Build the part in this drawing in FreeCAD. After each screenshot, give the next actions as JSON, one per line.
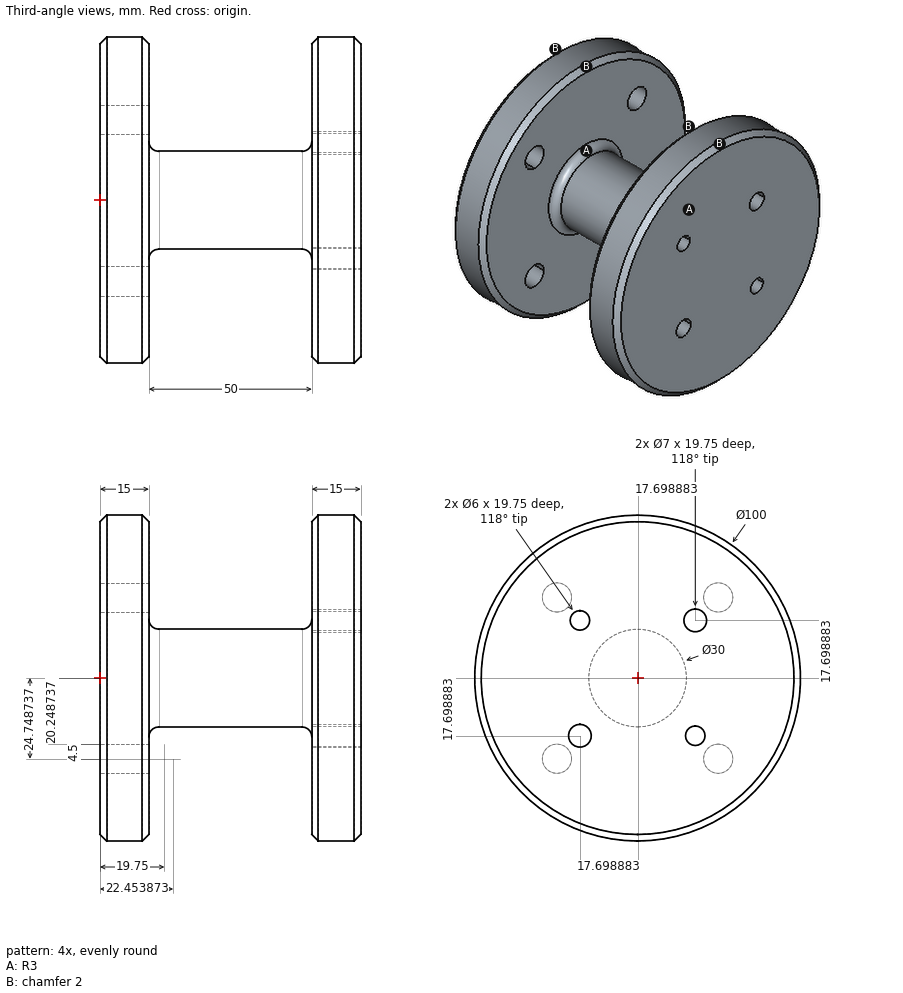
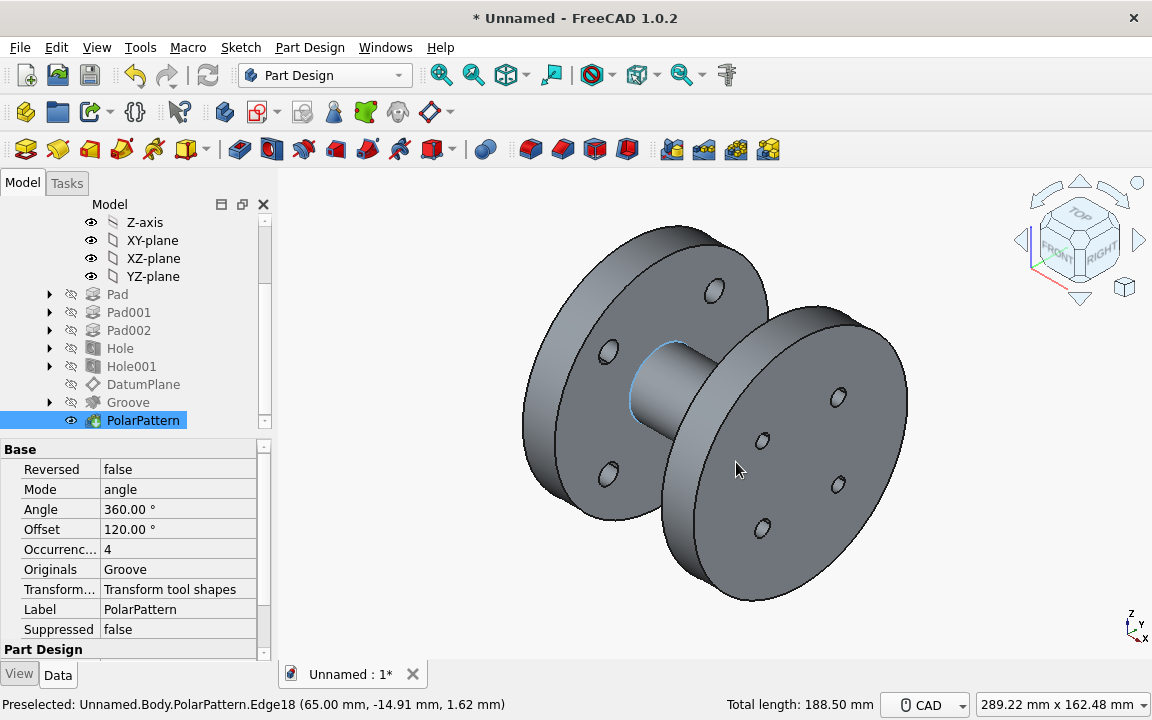
{"action": "left_click", "coordinate": [532, 150]}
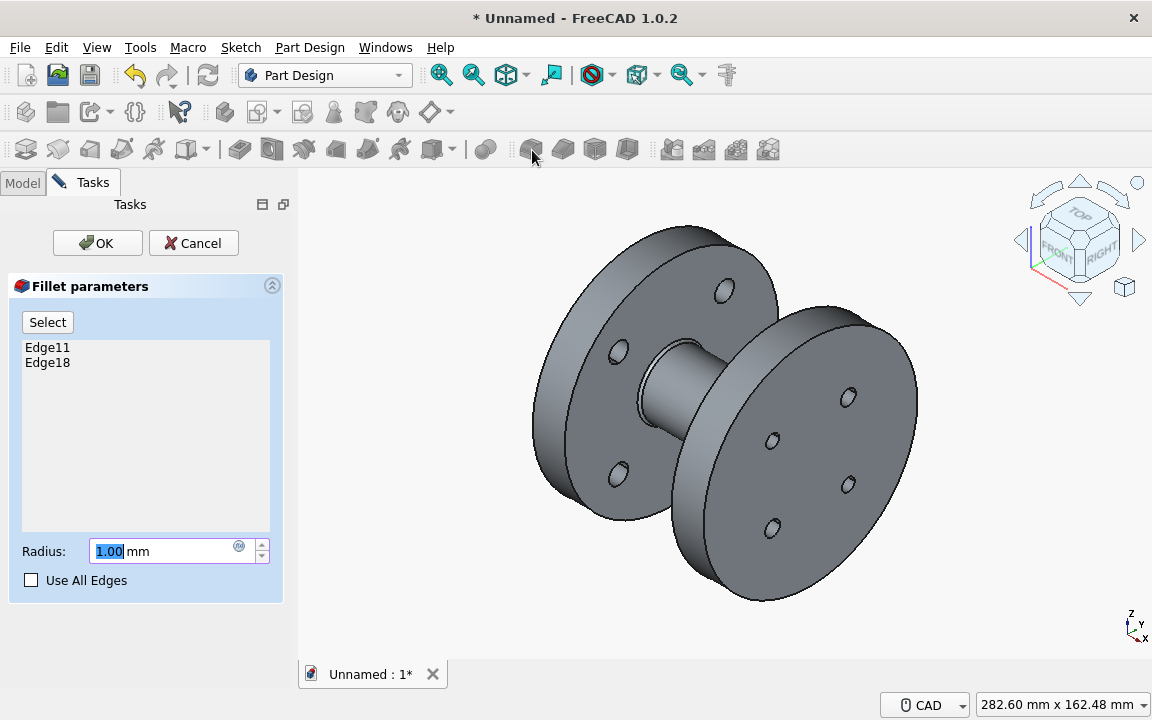
{"action": "type", "text": "3"}
{"action": "key", "text": "Tab"}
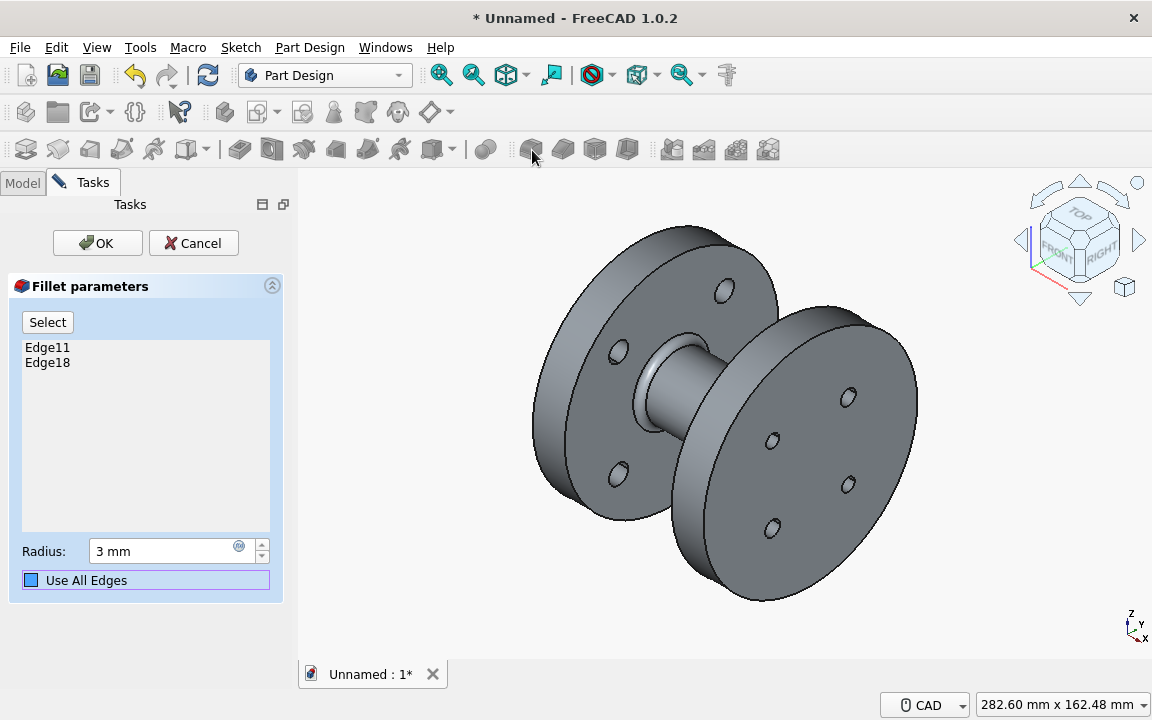
{"action": "left_click", "coordinate": [98, 243]}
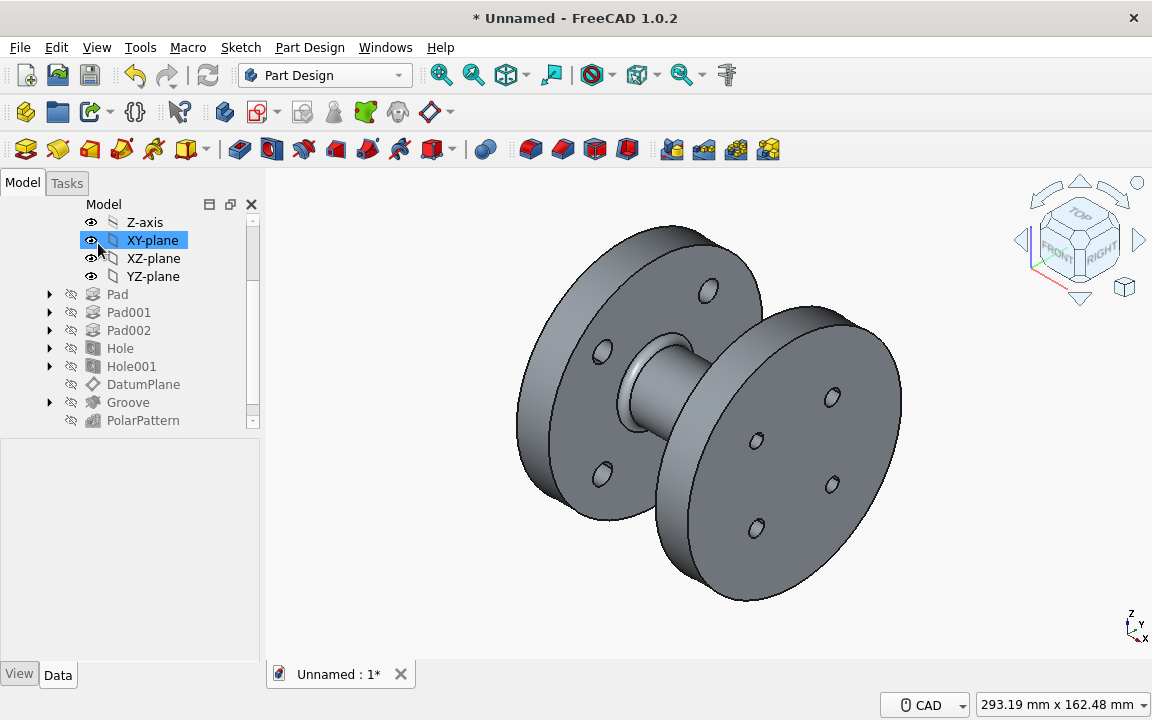
{"action": "left_click", "coordinate": [549, 443]}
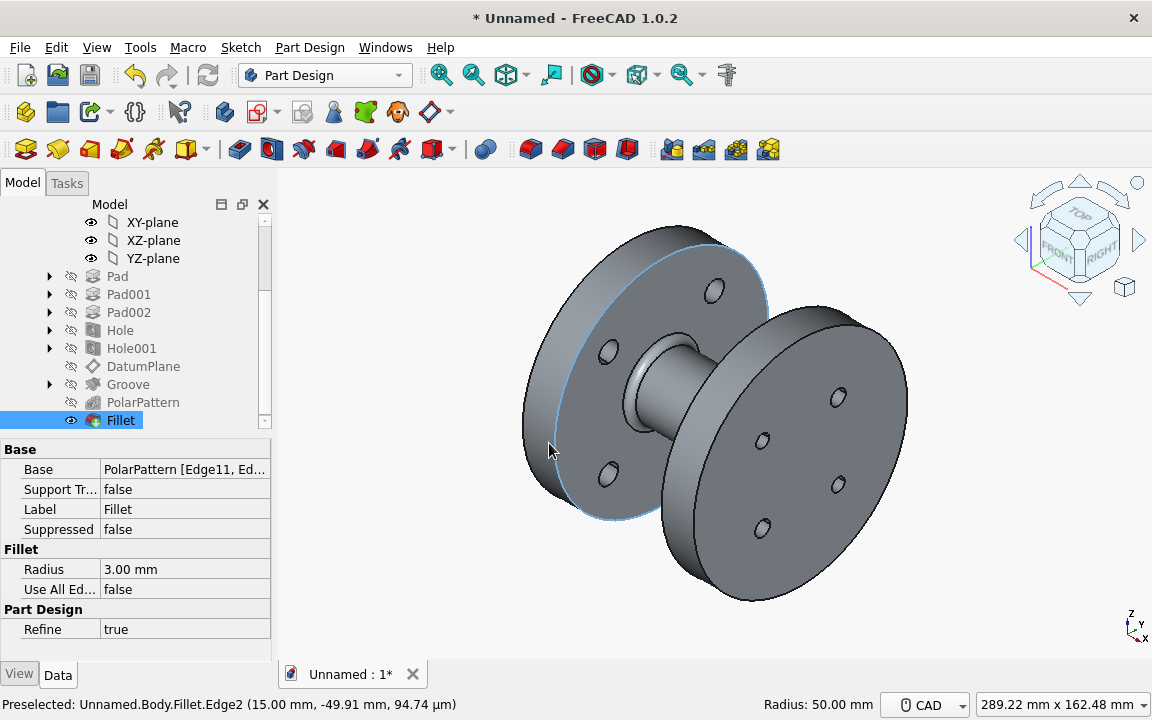
{"action": "left_click", "coordinate": [694, 524], "text": "ctrl"}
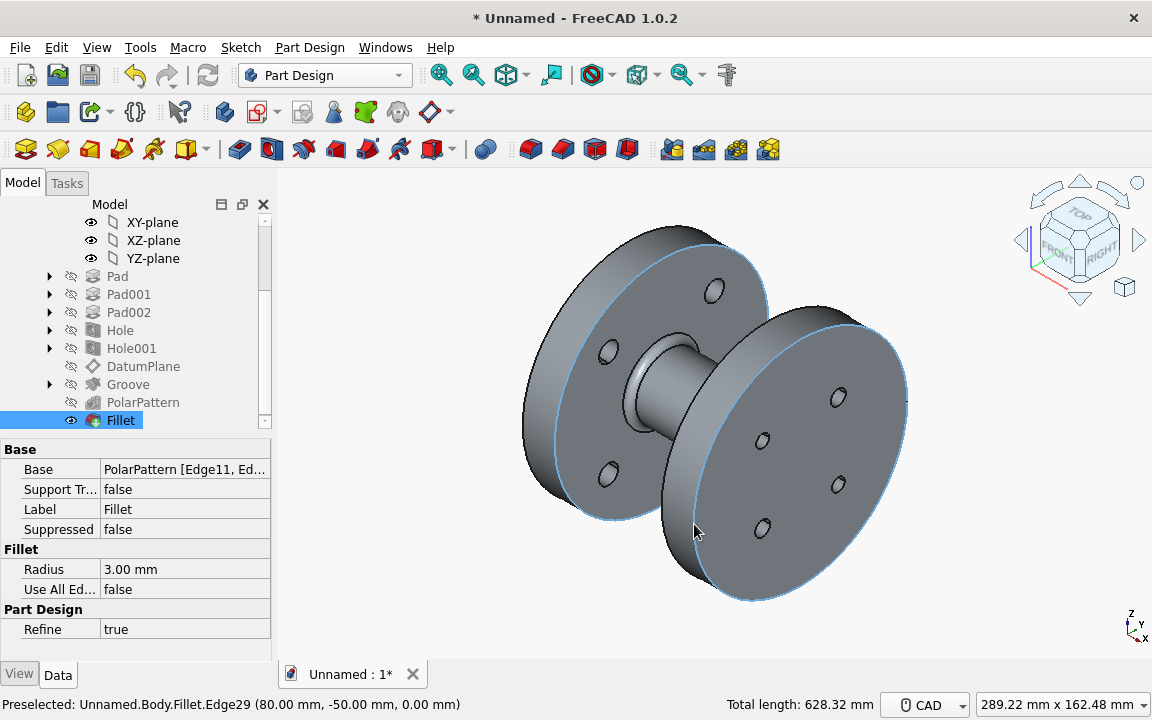
{"action": "key", "text": "2"}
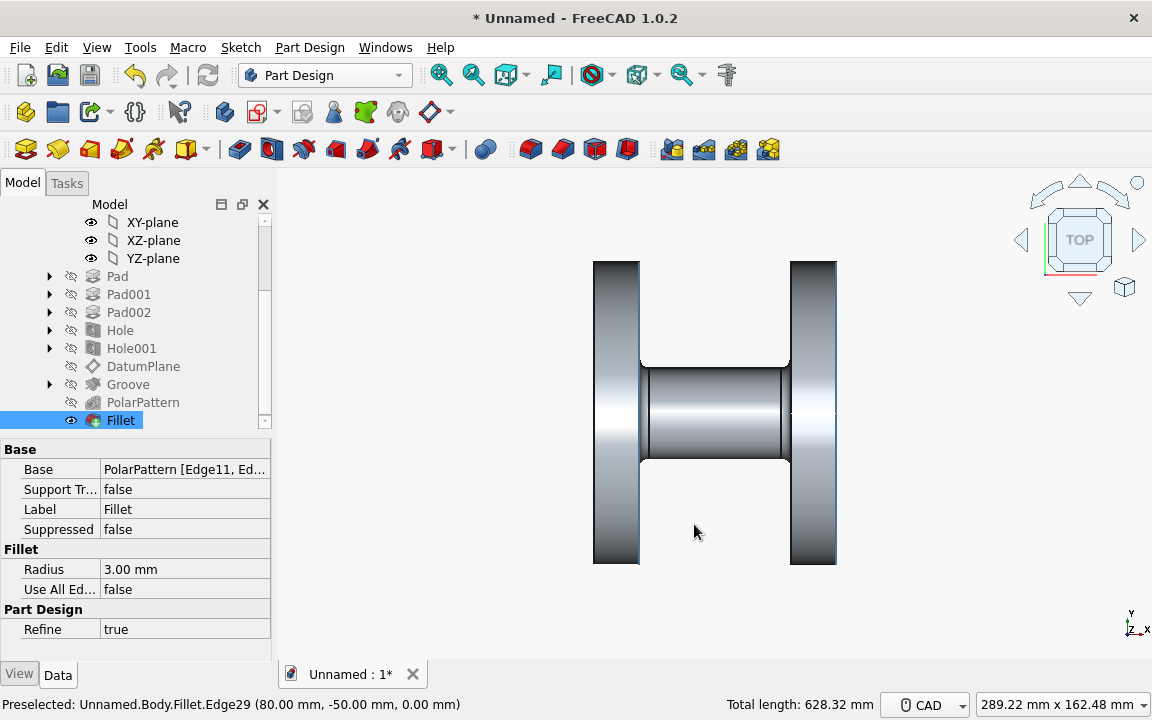
{"action": "left_click", "coordinate": [594, 535], "text": "ctrl"}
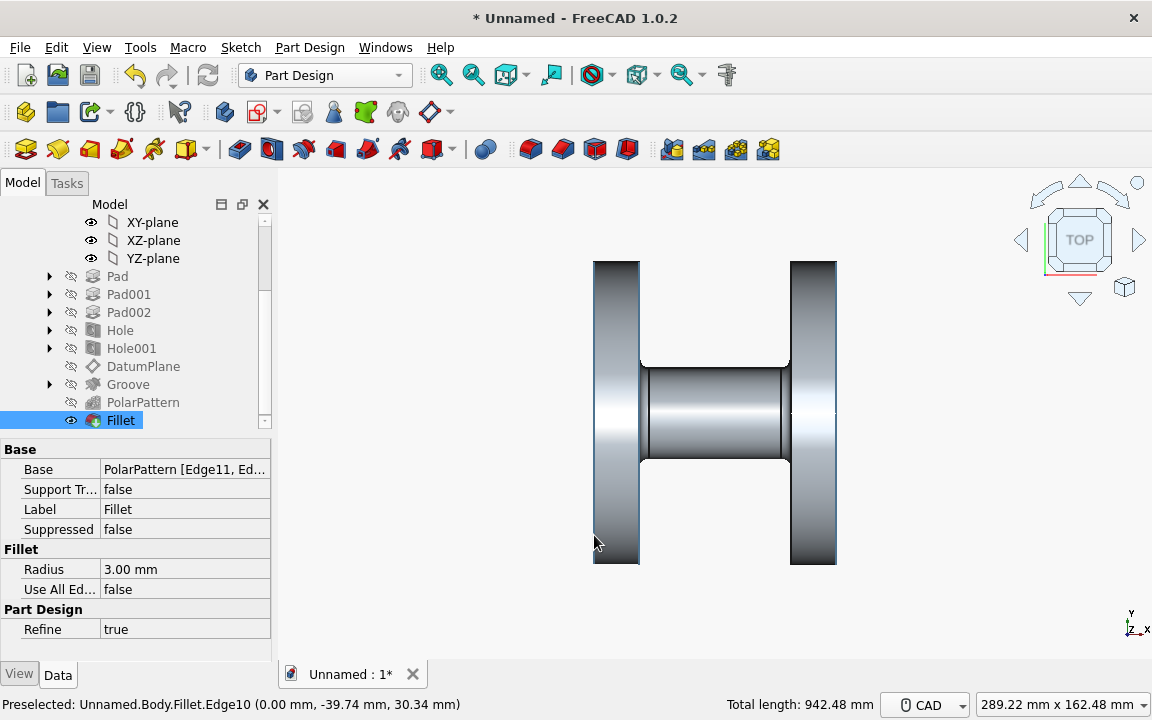
{"action": "left_click", "coordinate": [791, 535], "text": "ctrl"}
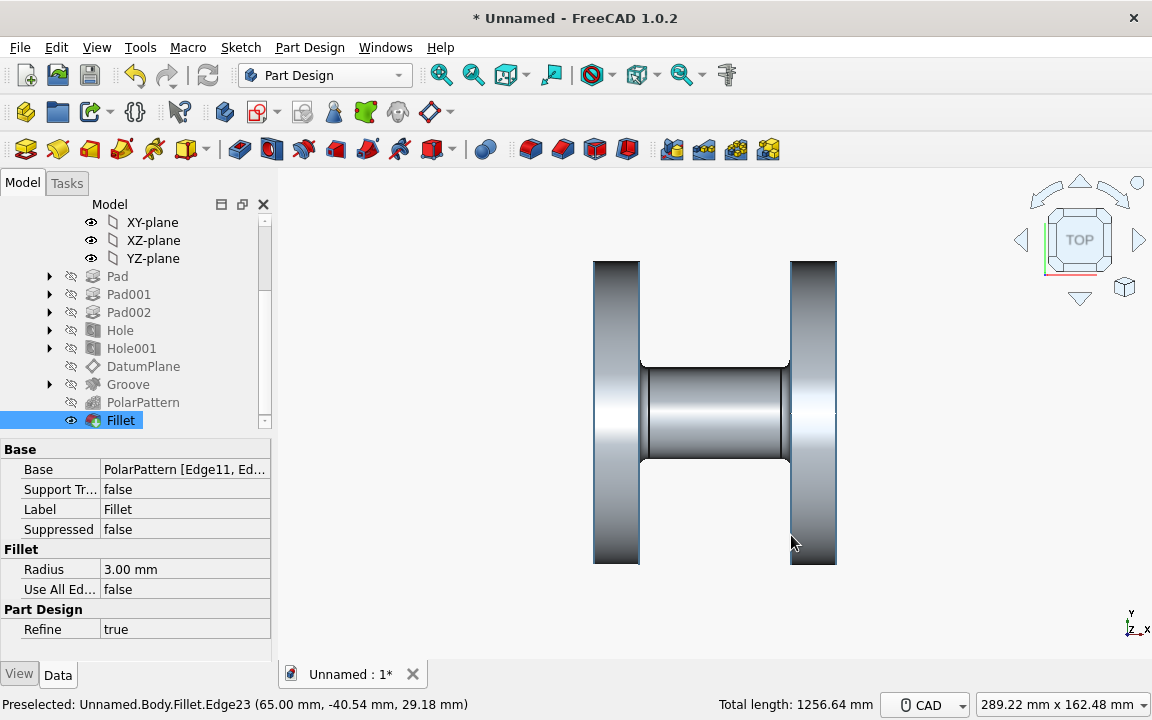
{"action": "left_click", "coordinate": [564, 150]}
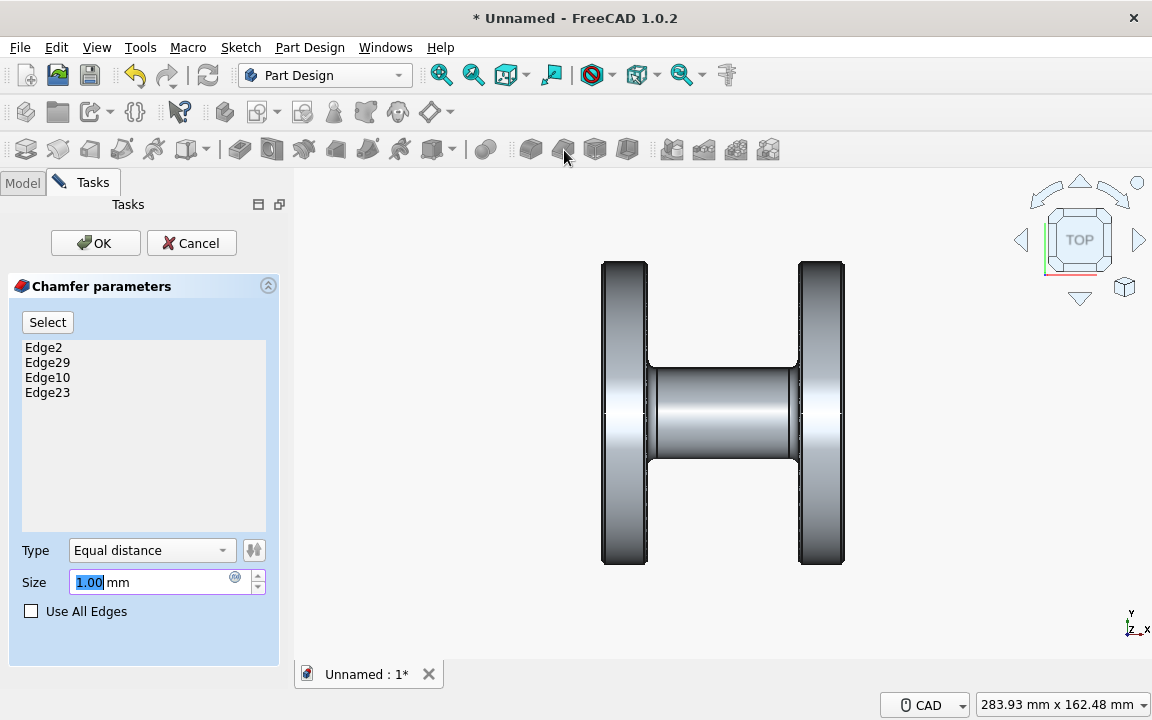
{"action": "type", "text": "2"}
{"action": "key", "text": "Tab"}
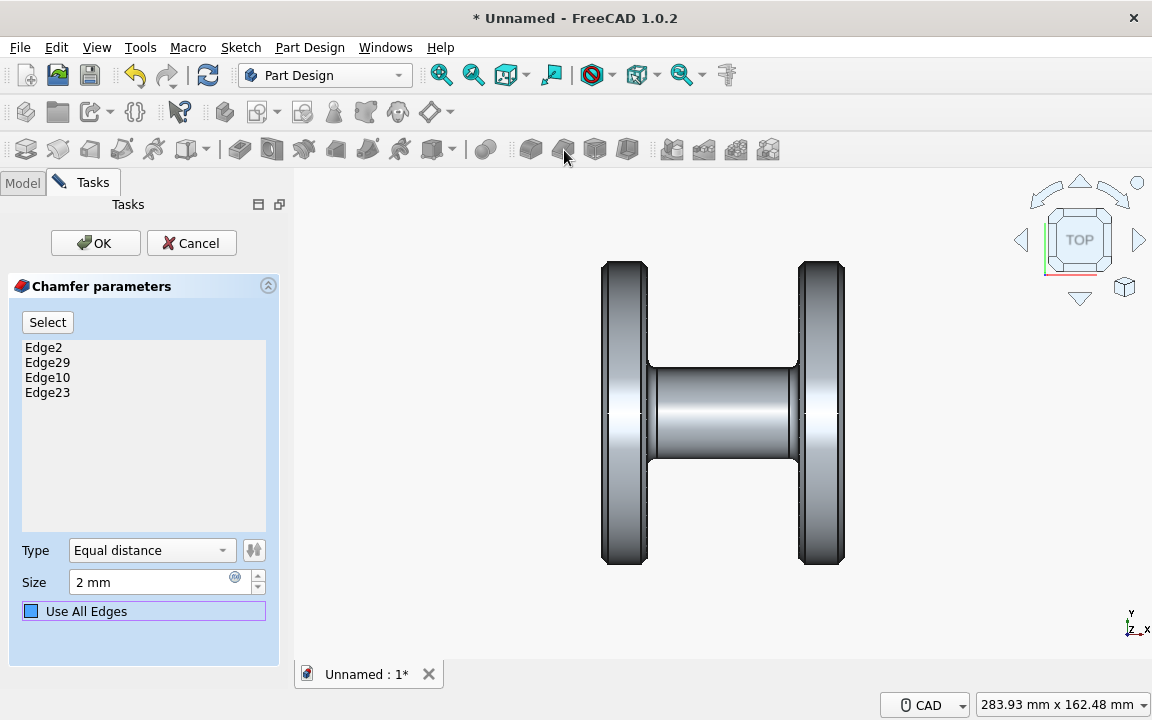
{"action": "left_click", "coordinate": [96, 243]}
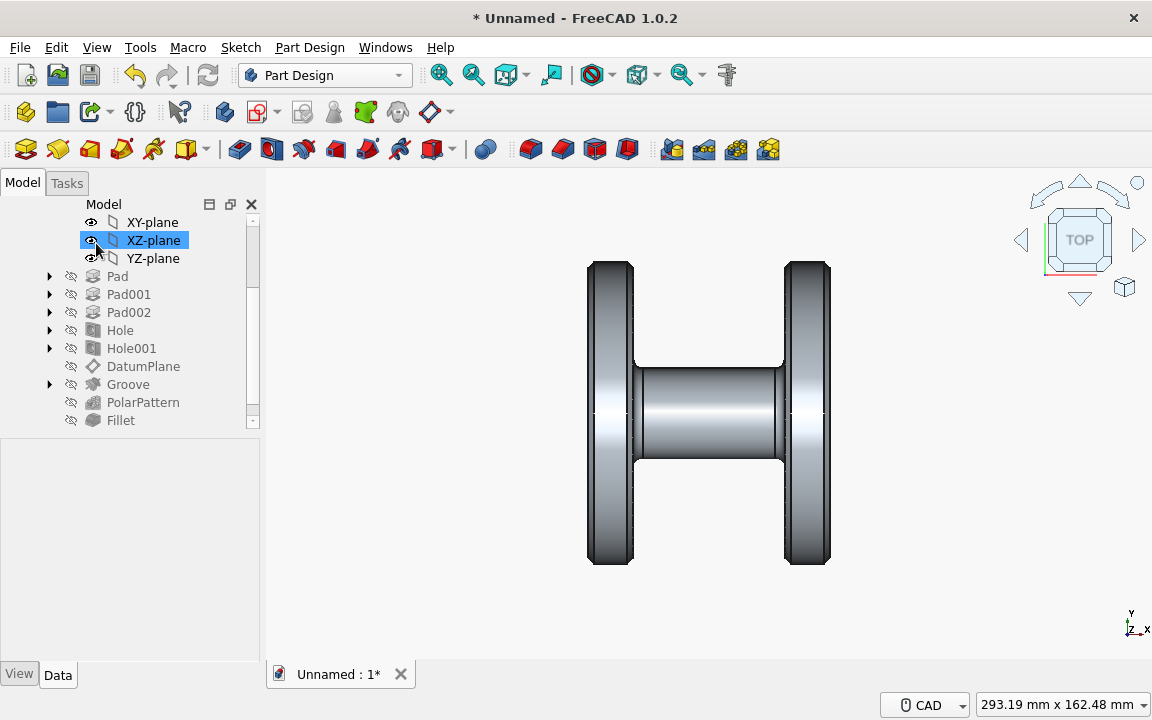
{"action": "key", "text": "0"}